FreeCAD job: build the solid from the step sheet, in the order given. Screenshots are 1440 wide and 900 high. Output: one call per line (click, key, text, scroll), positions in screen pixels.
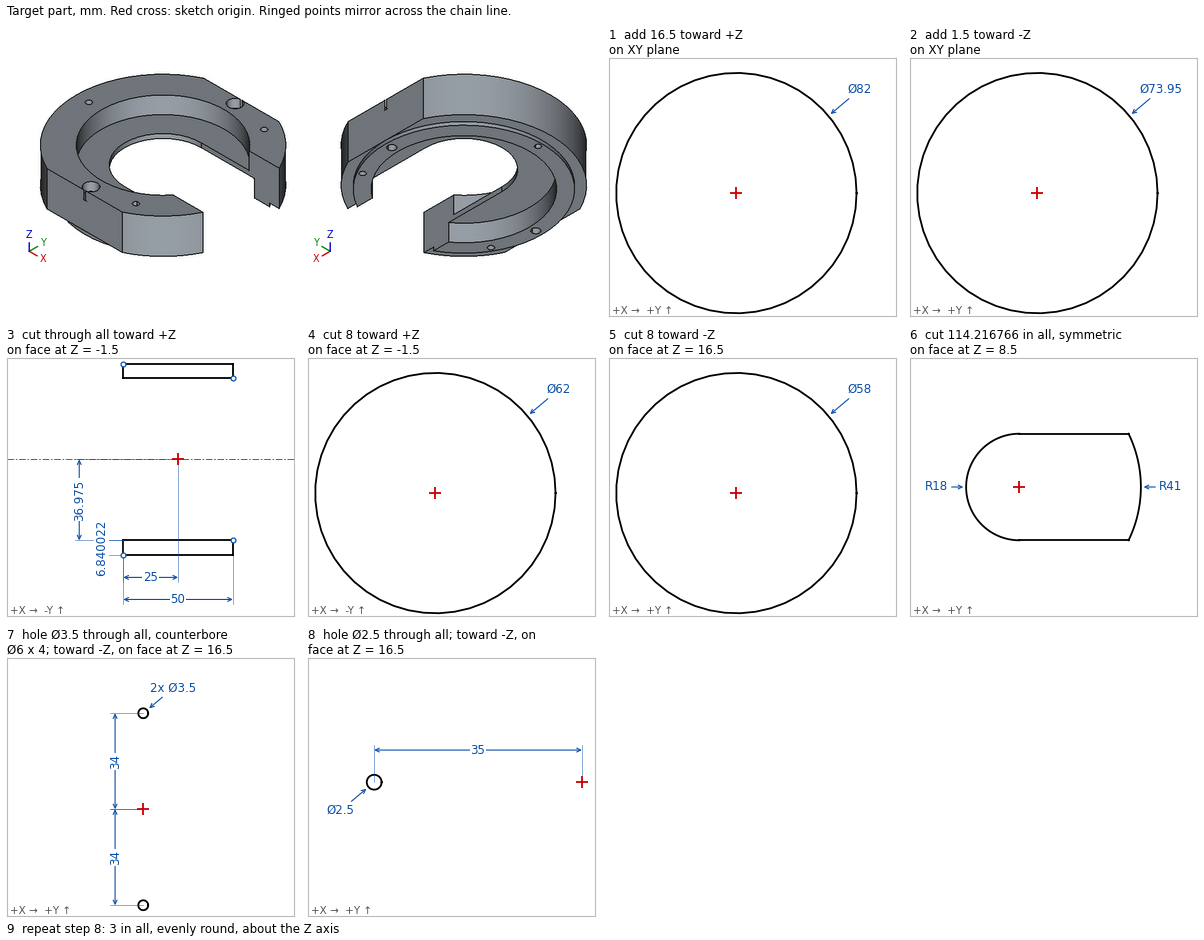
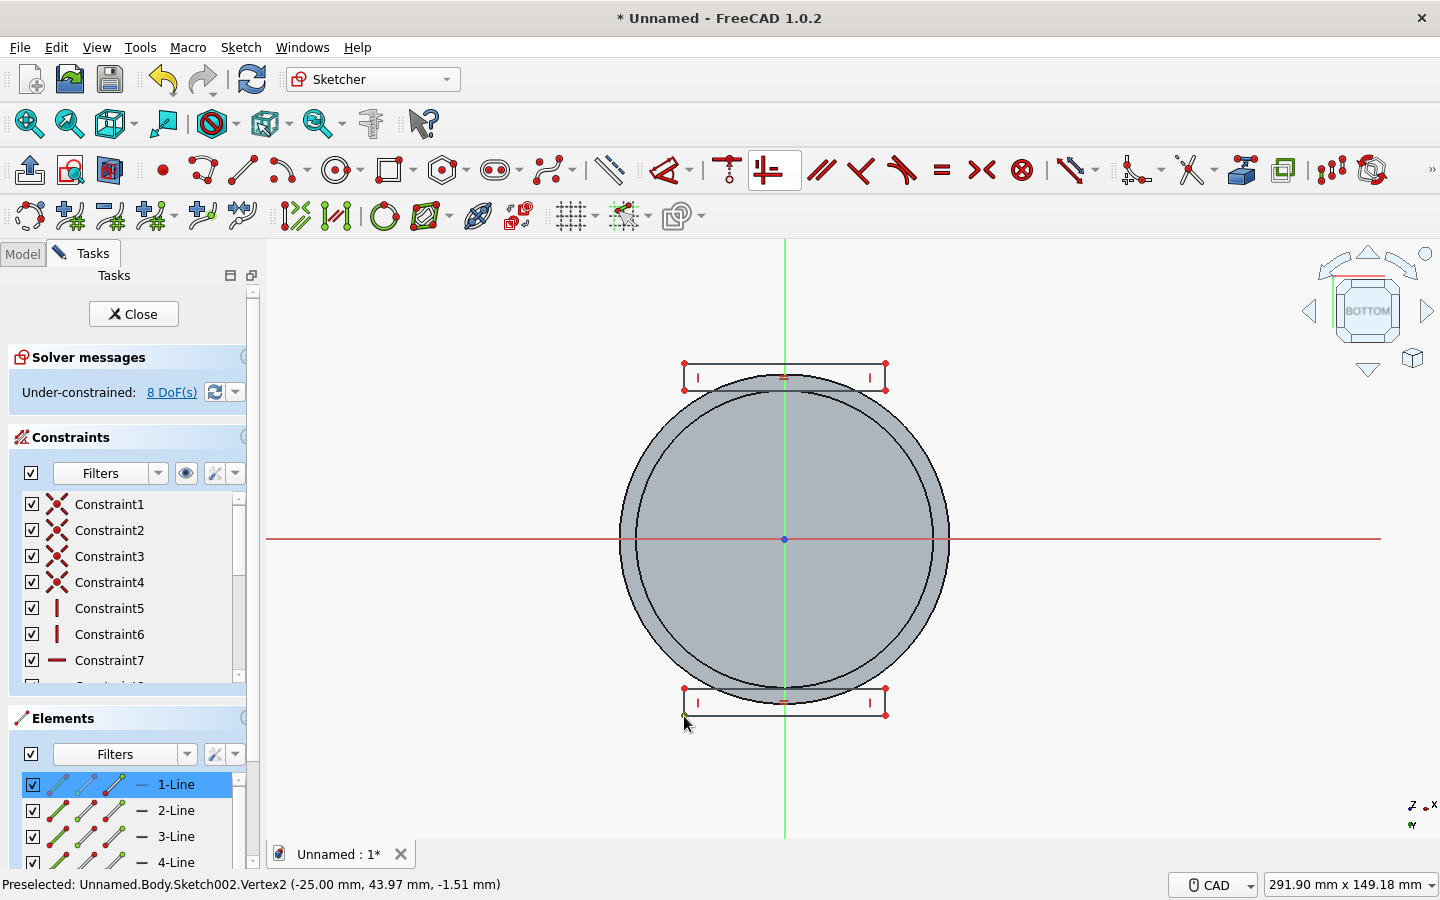
click(684, 364)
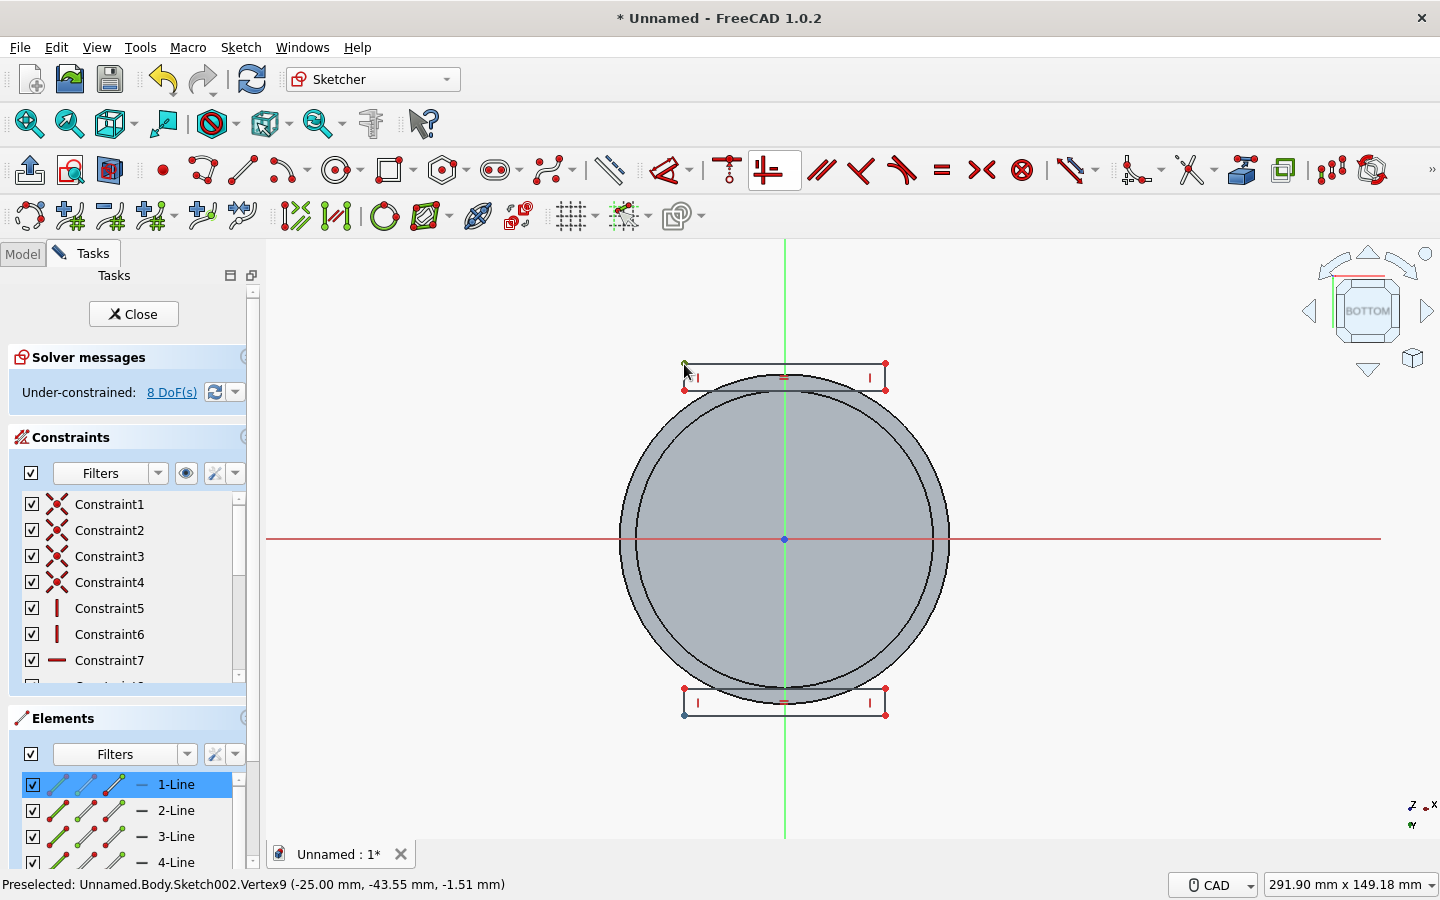
click(364, 539)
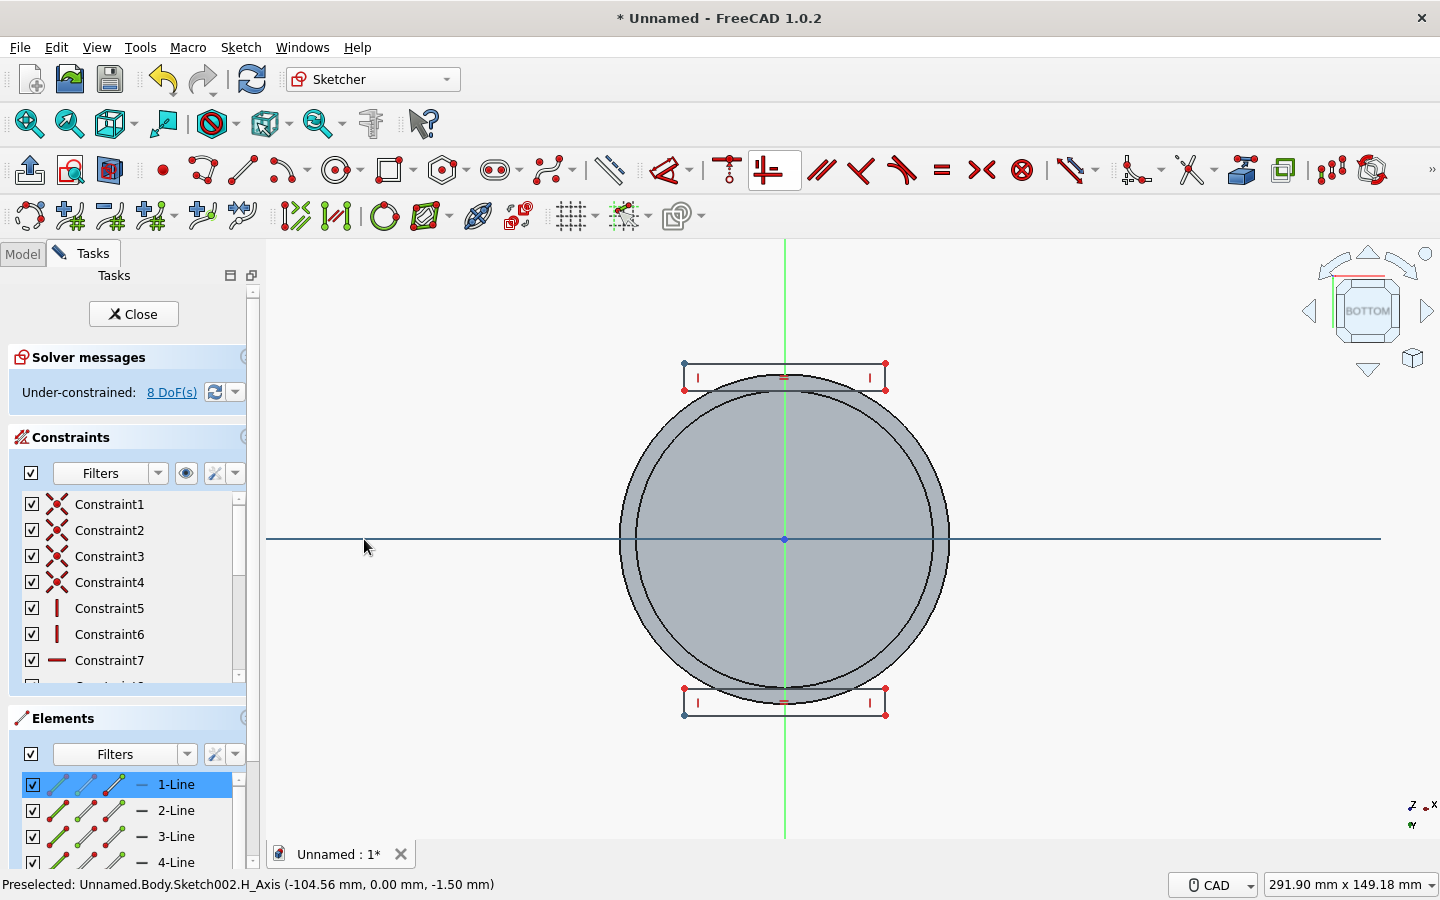
click(982, 170)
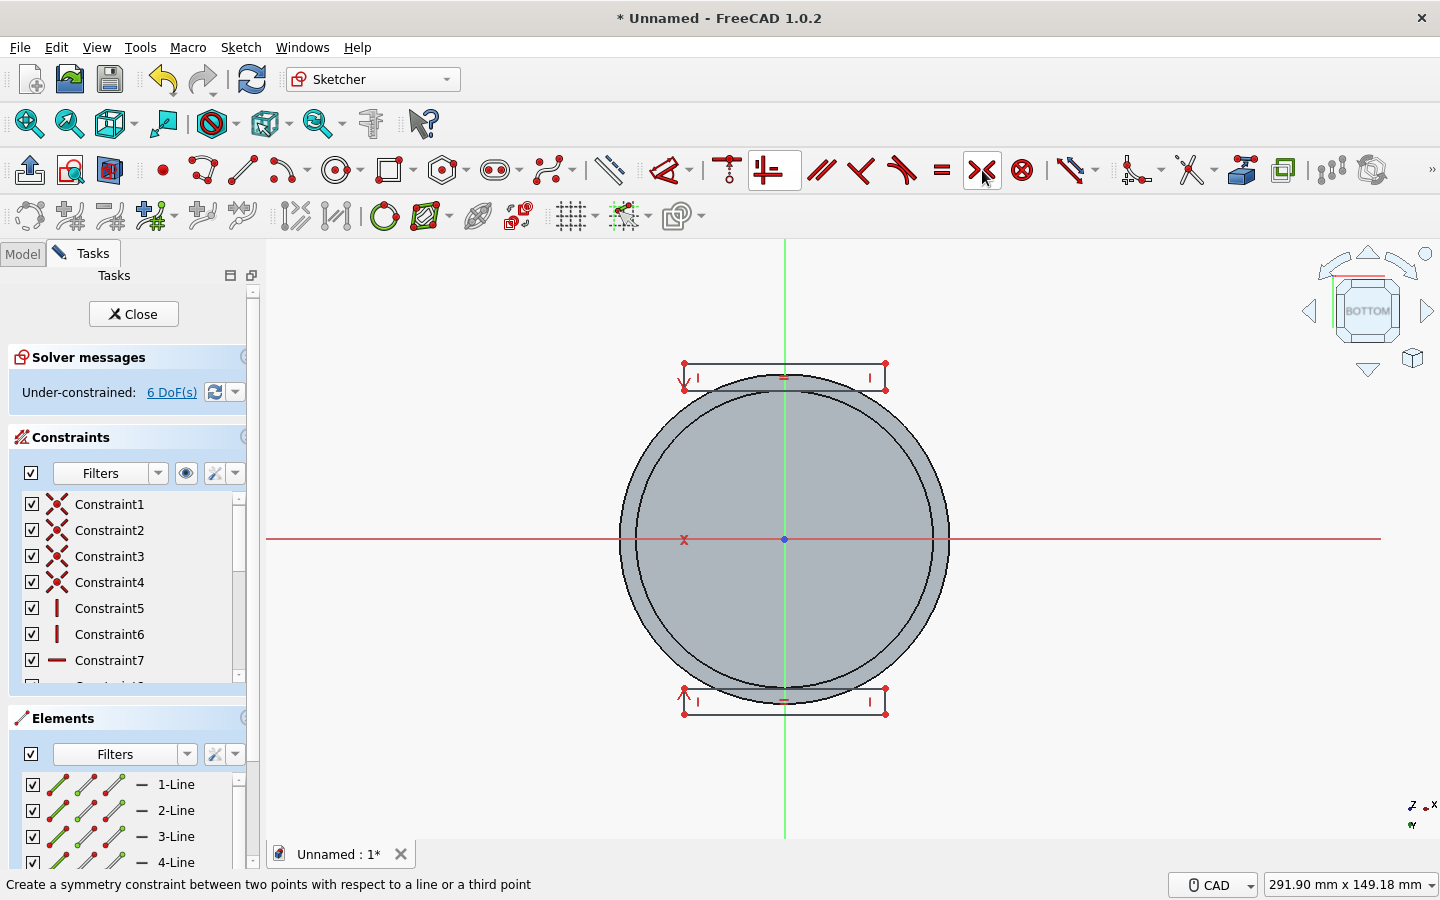
click(885, 689)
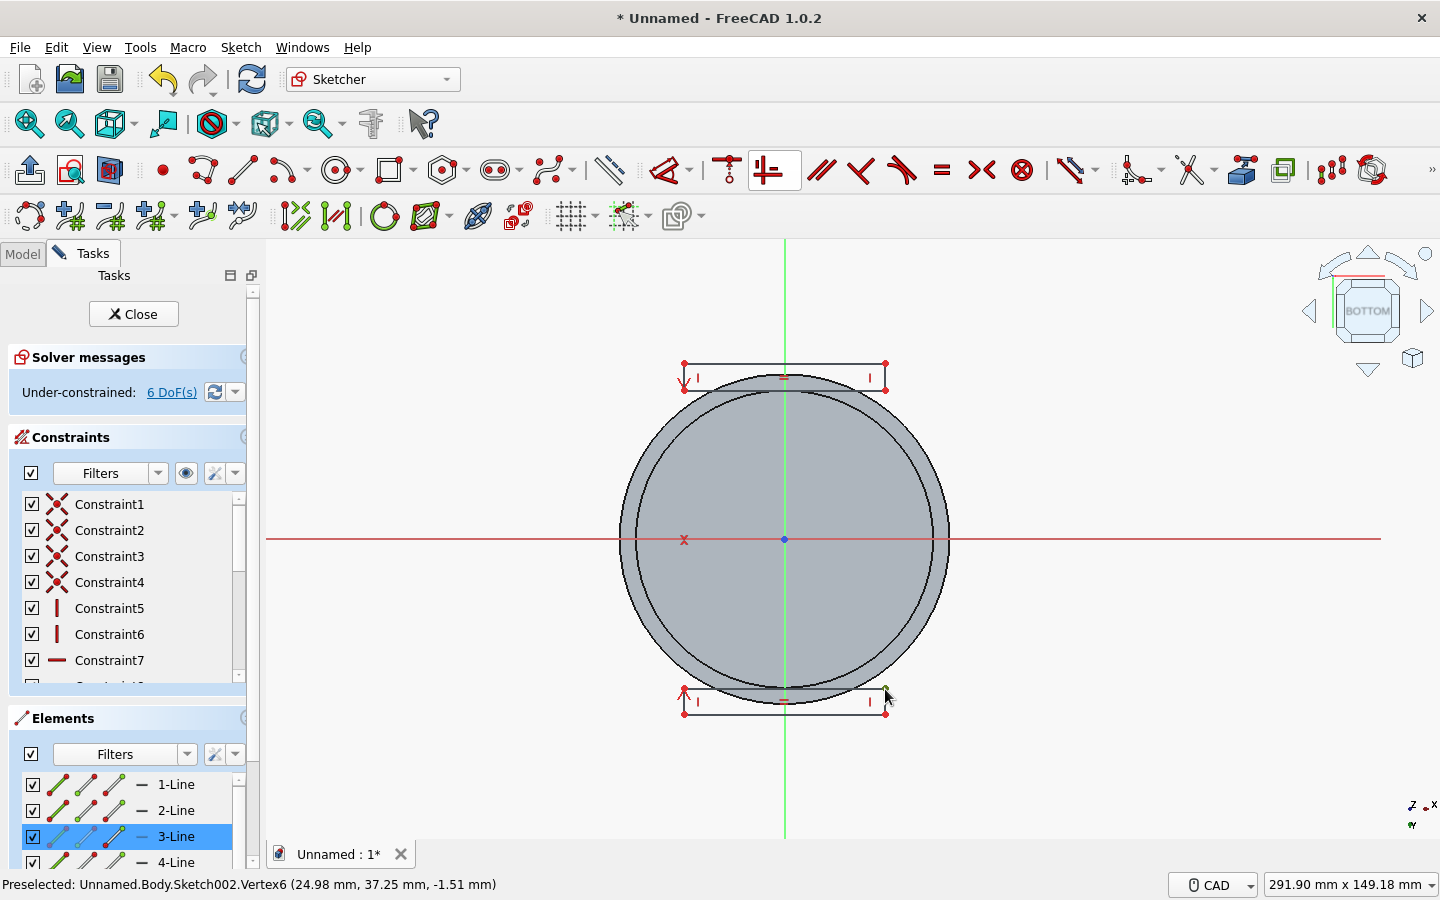
click(885, 391)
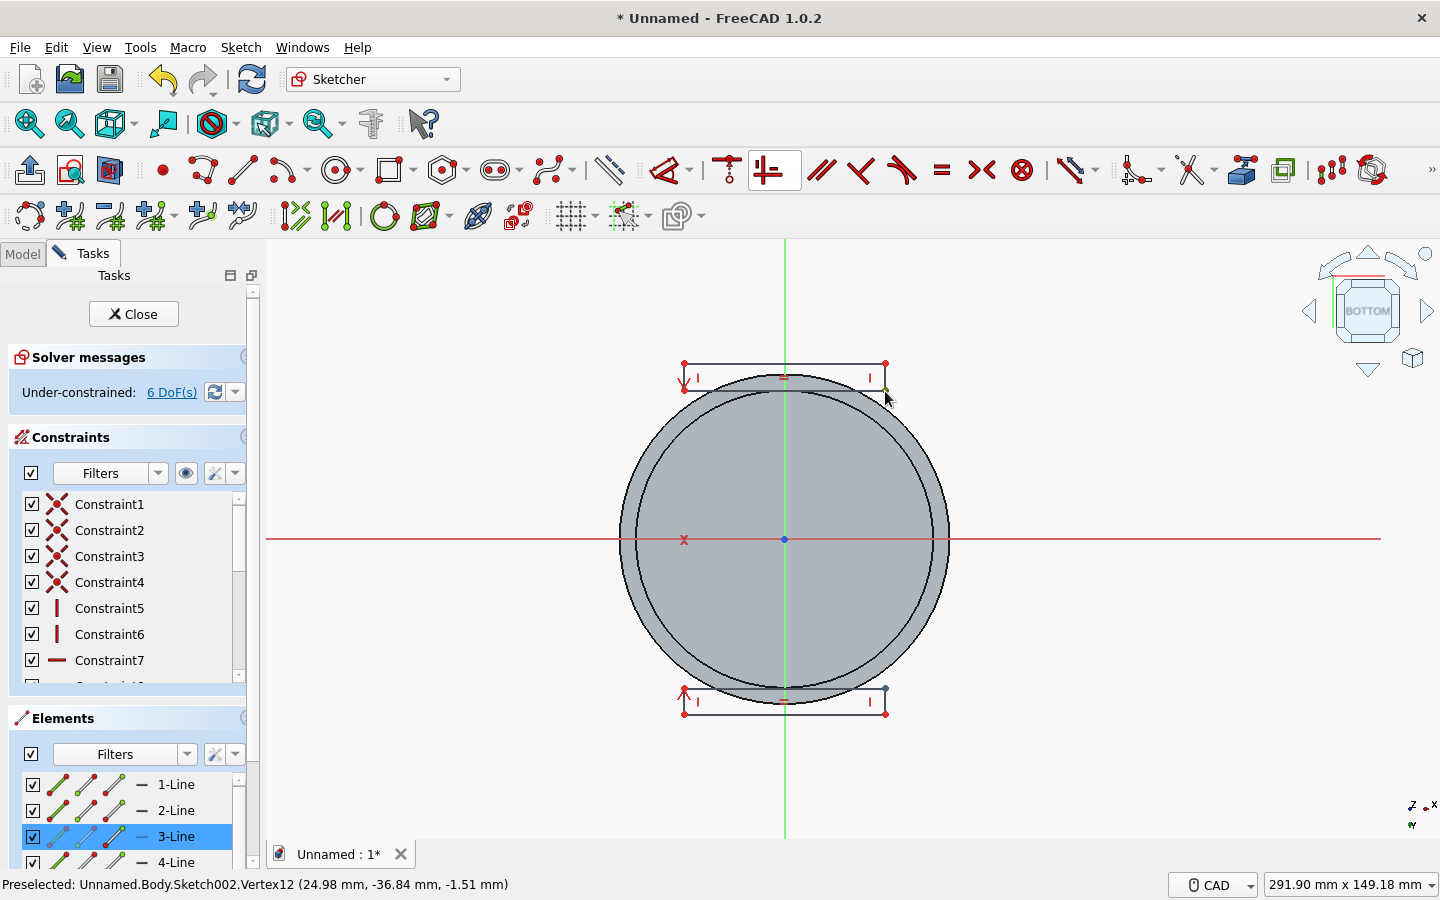
click(364, 539)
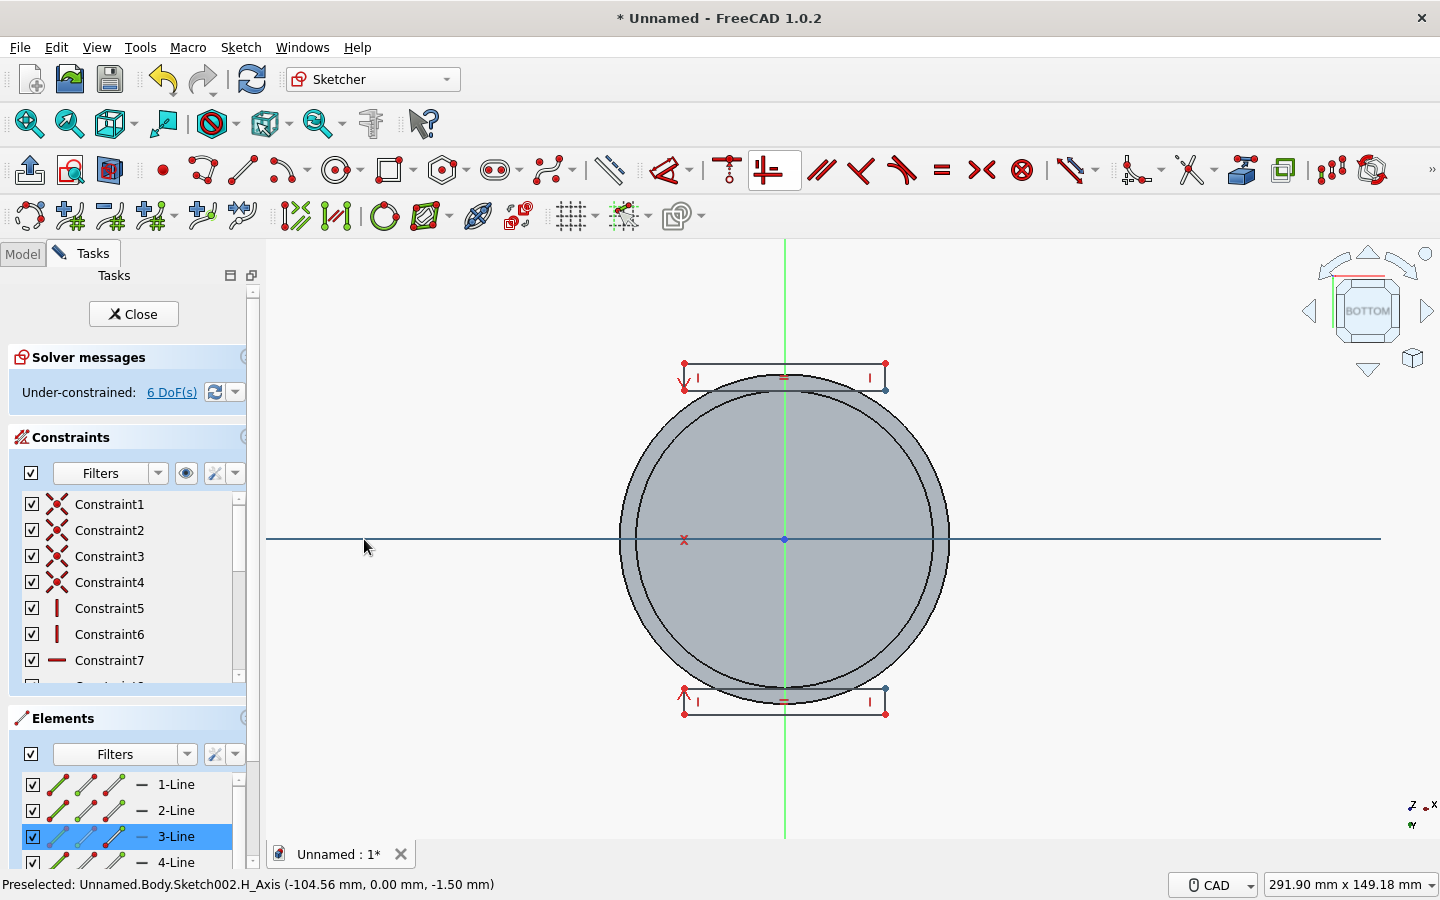
click(982, 170)